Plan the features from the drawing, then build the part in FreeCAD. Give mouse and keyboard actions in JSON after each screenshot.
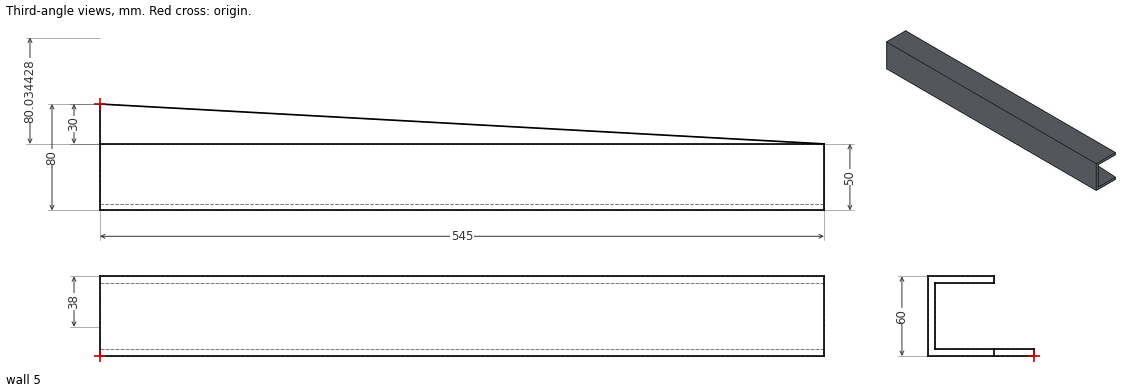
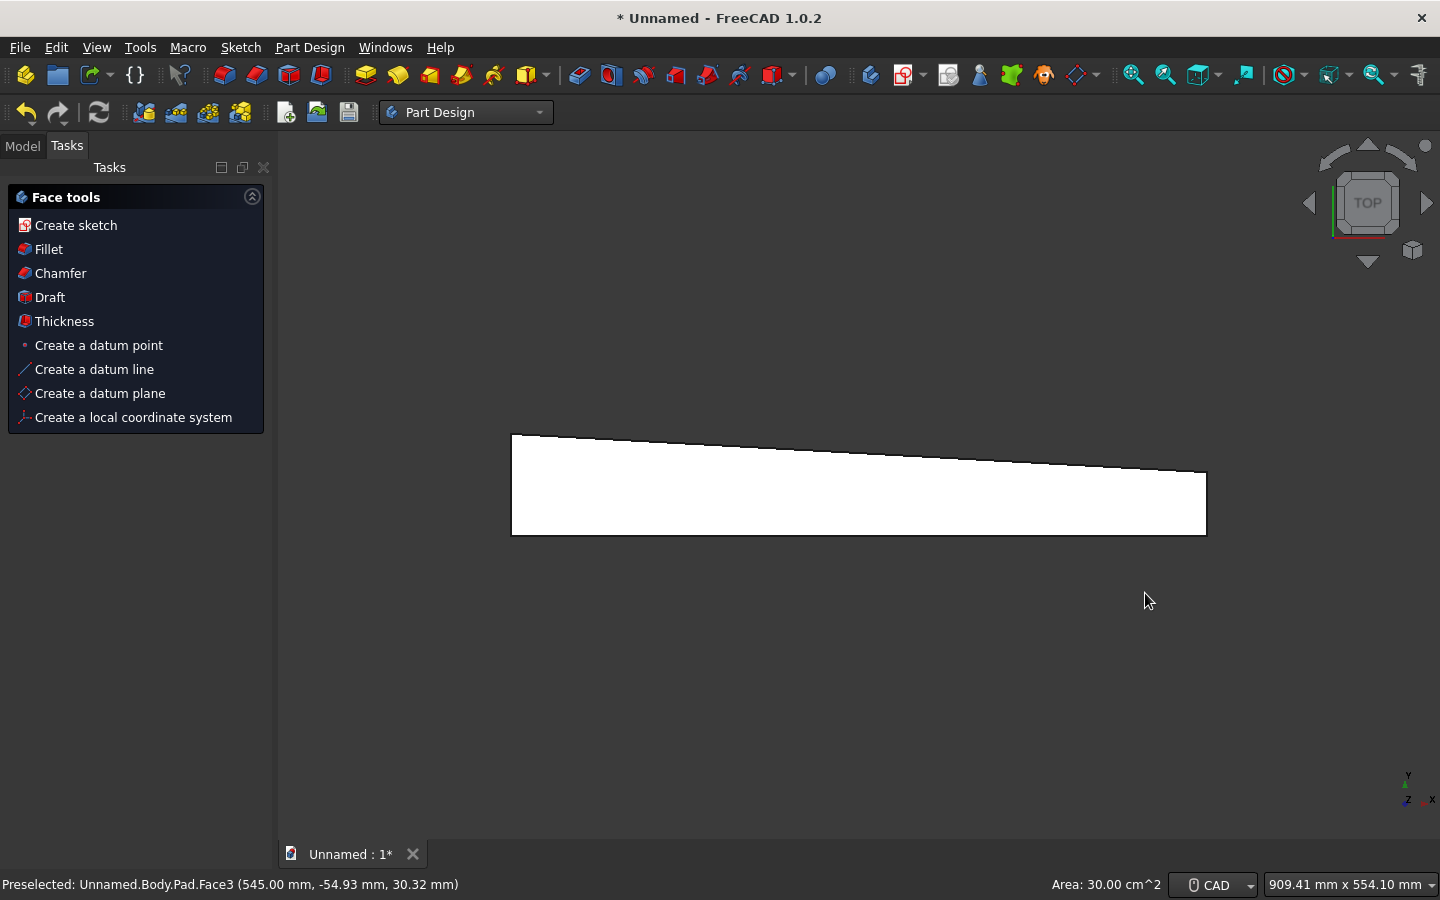
{"action": "key", "text": "1"}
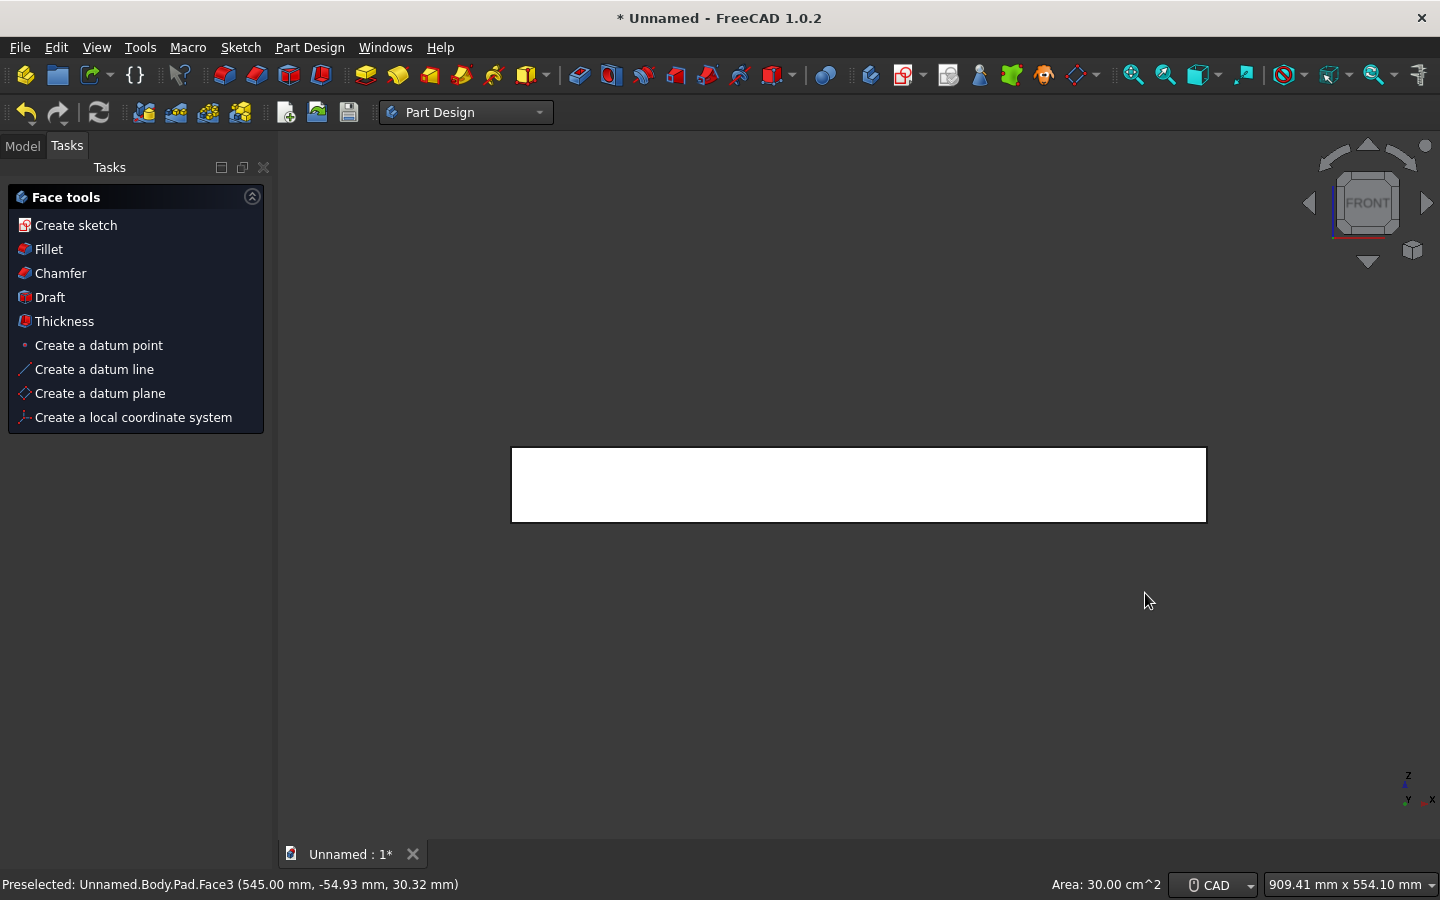
{"action": "key", "text": "3"}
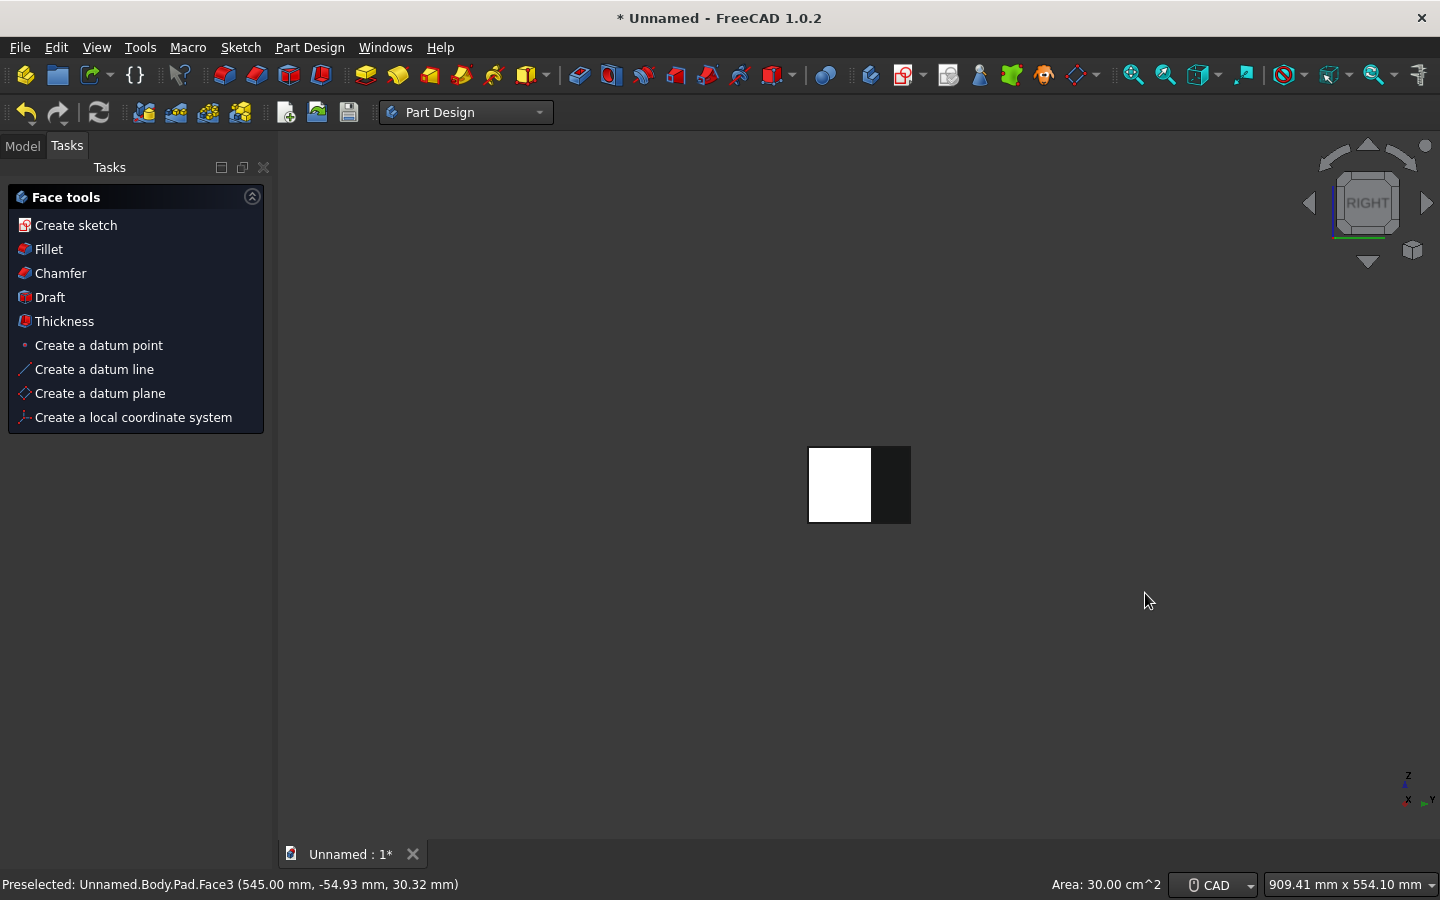
{"action": "left_click", "coordinate": [1134, 76]}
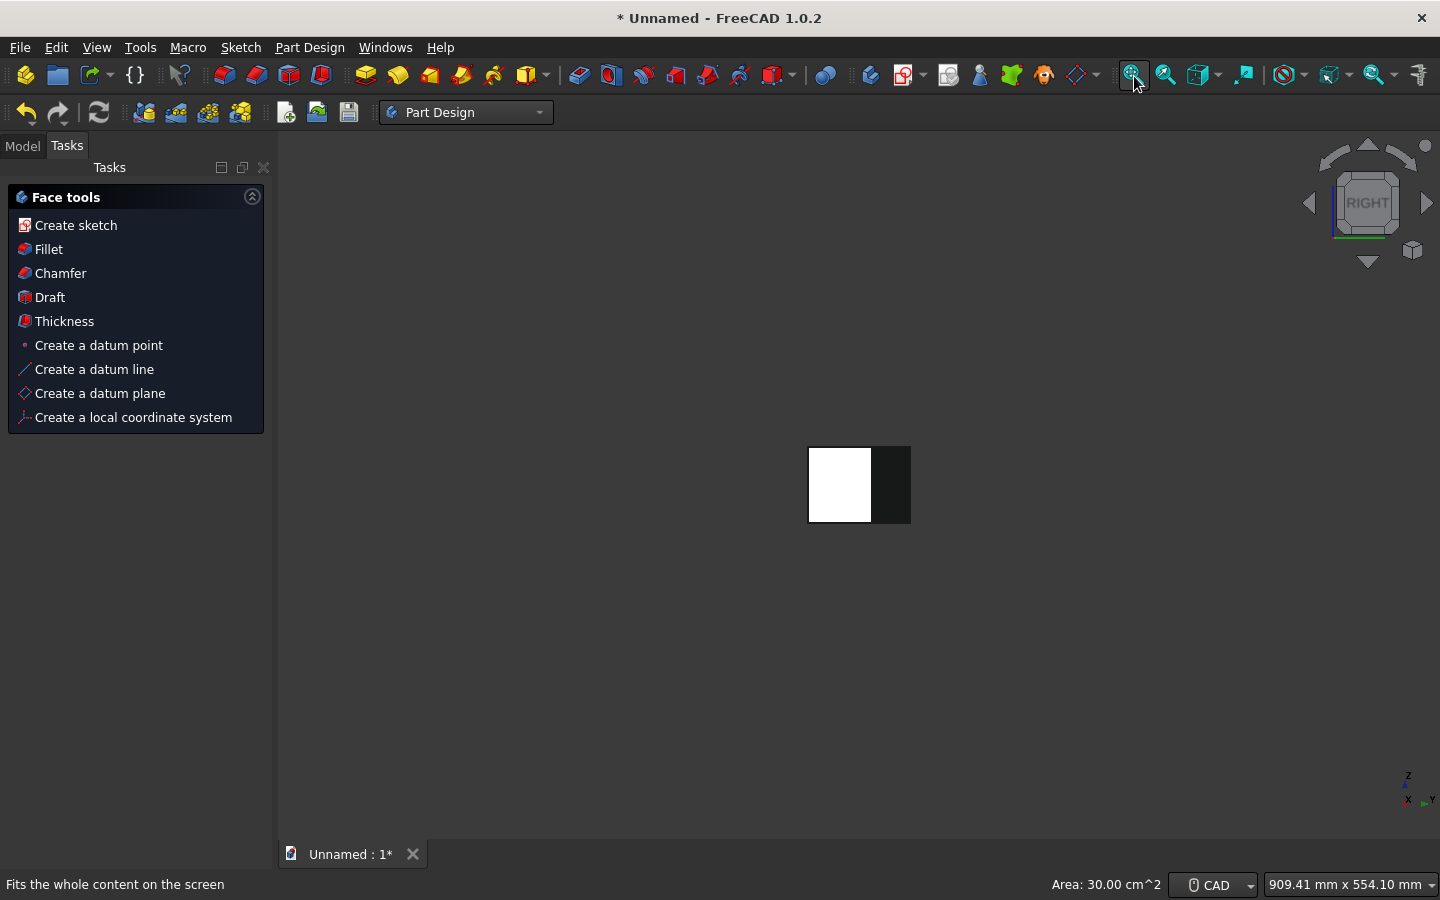
{"action": "left_click", "coordinate": [880, 484], "text": "ctrl"}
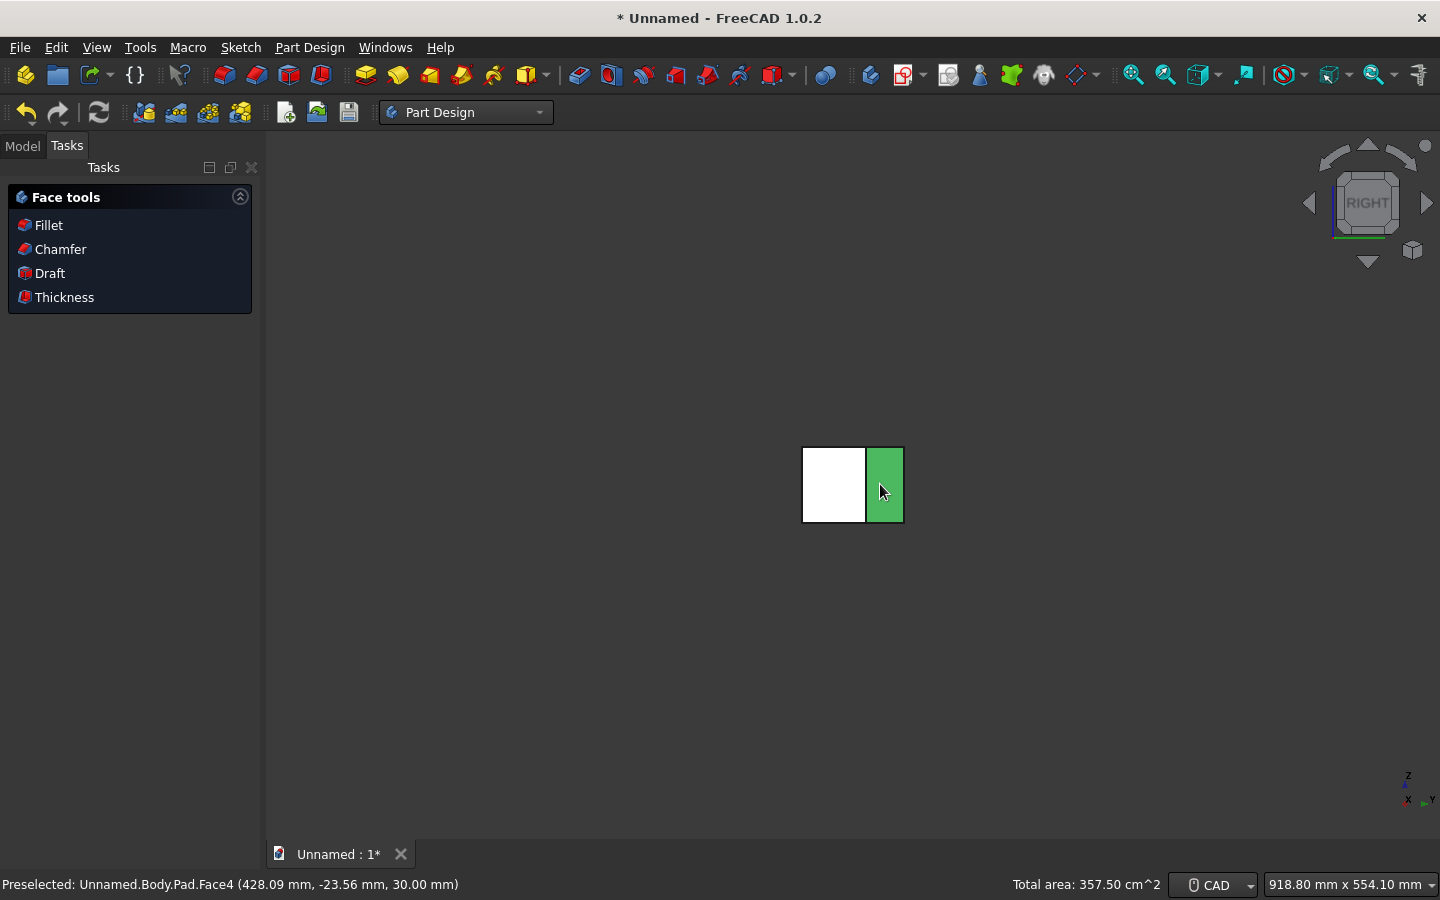
{"action": "key", "text": "5"}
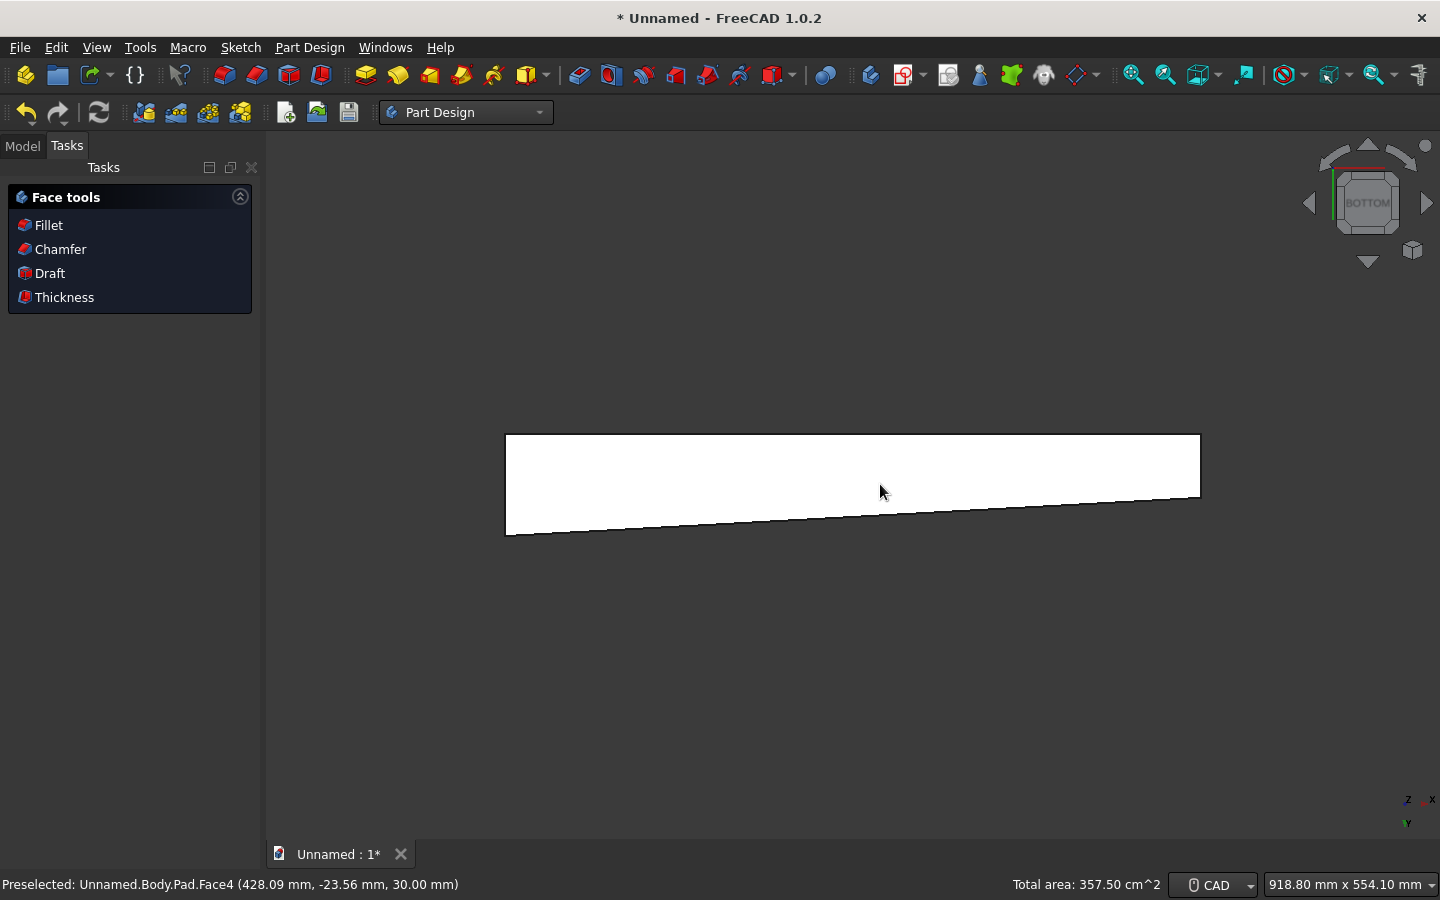
{"action": "key", "text": "4"}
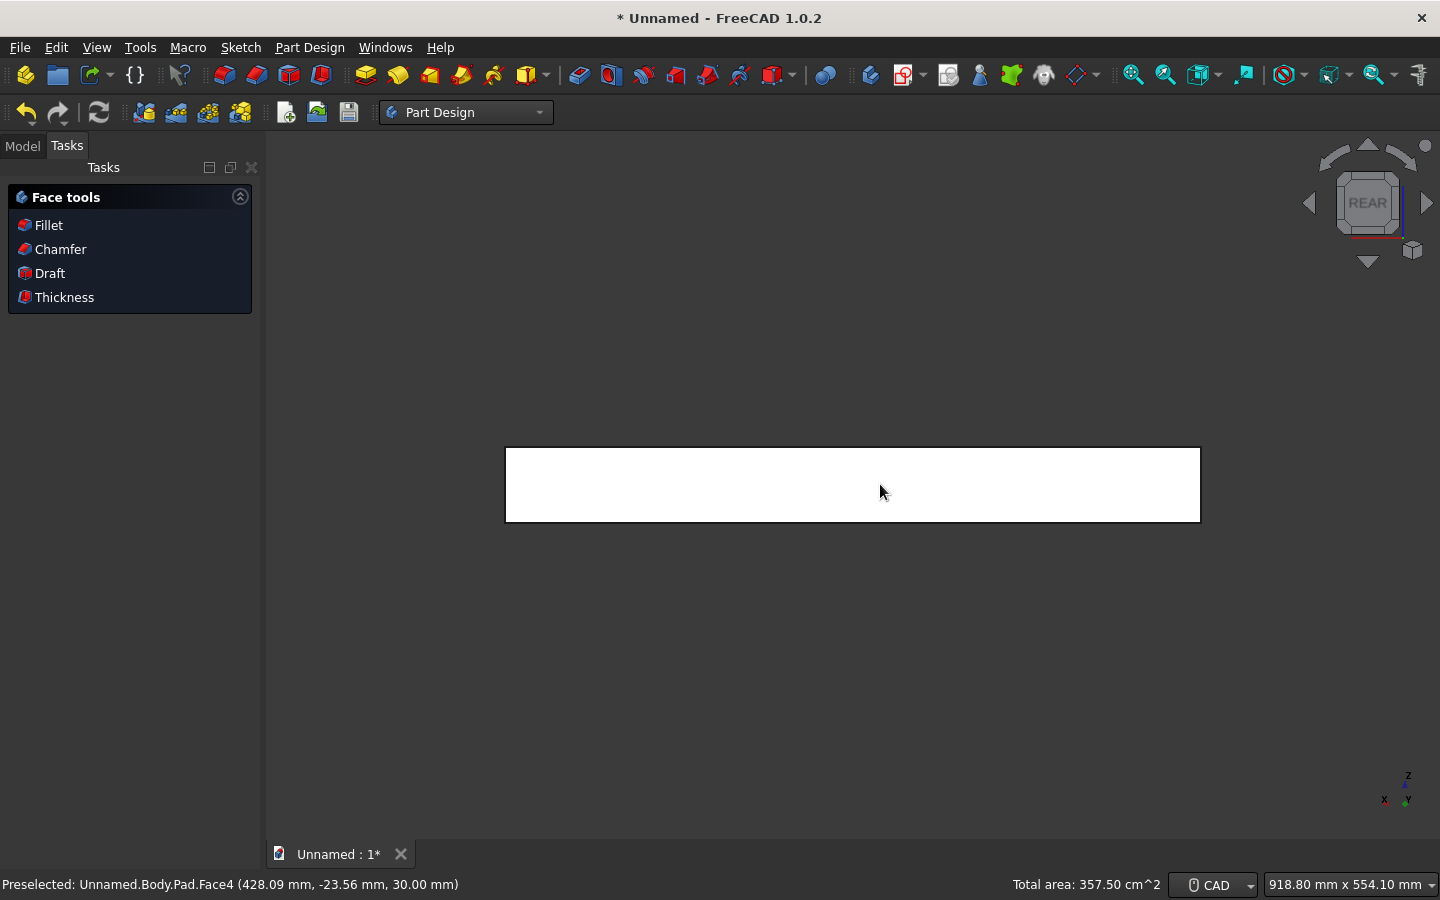
{"action": "key", "text": "6"}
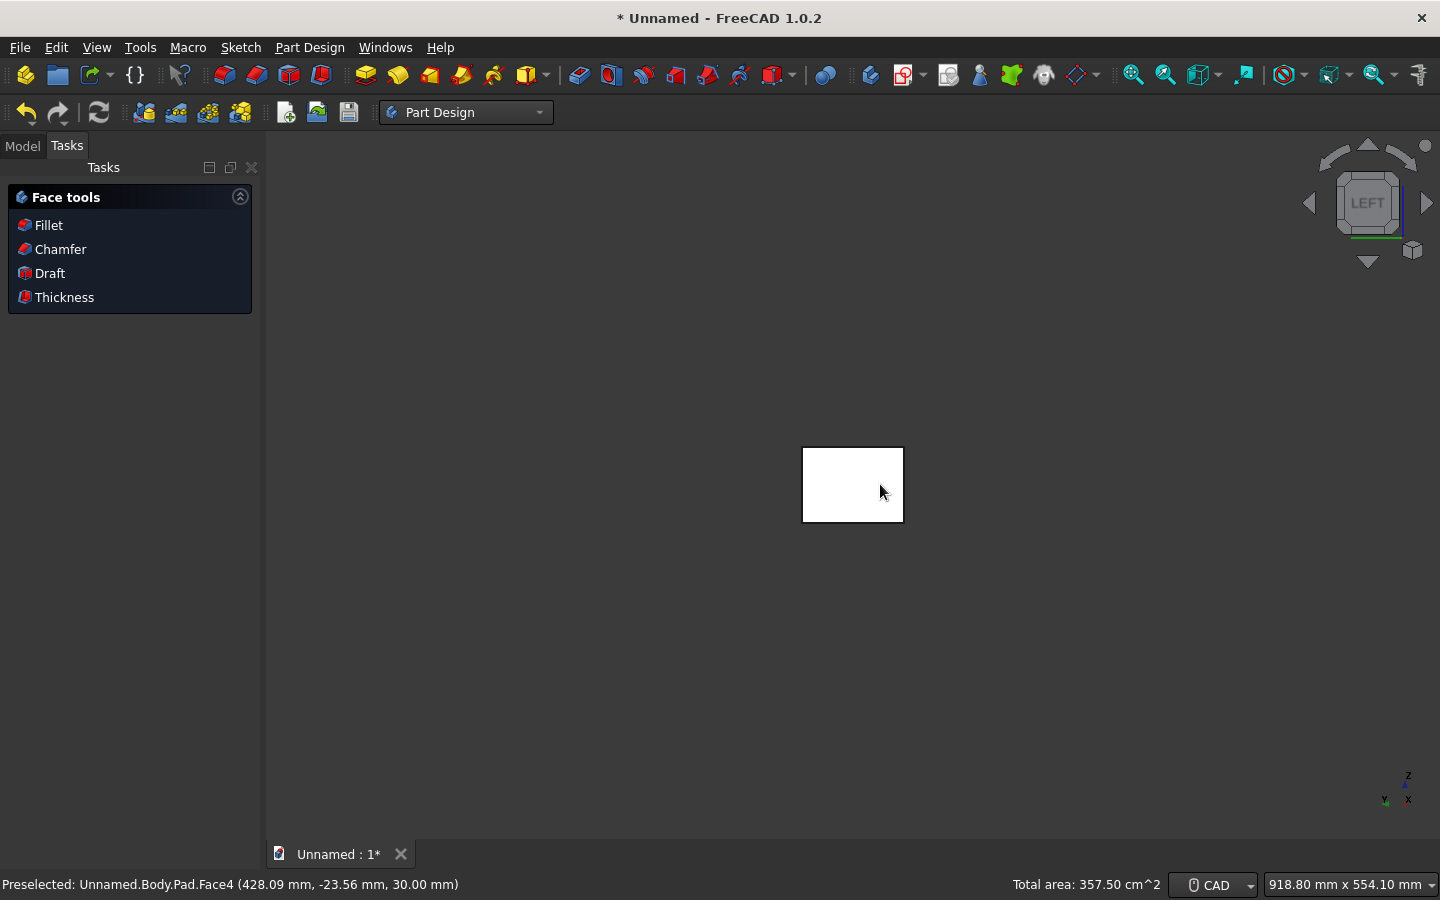
{"action": "key", "text": "v f"}